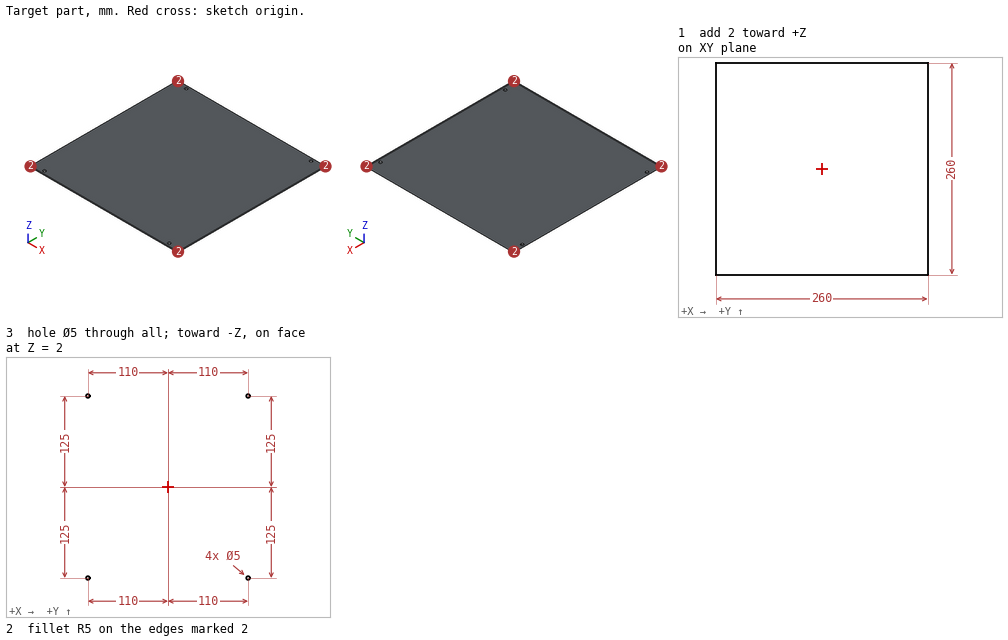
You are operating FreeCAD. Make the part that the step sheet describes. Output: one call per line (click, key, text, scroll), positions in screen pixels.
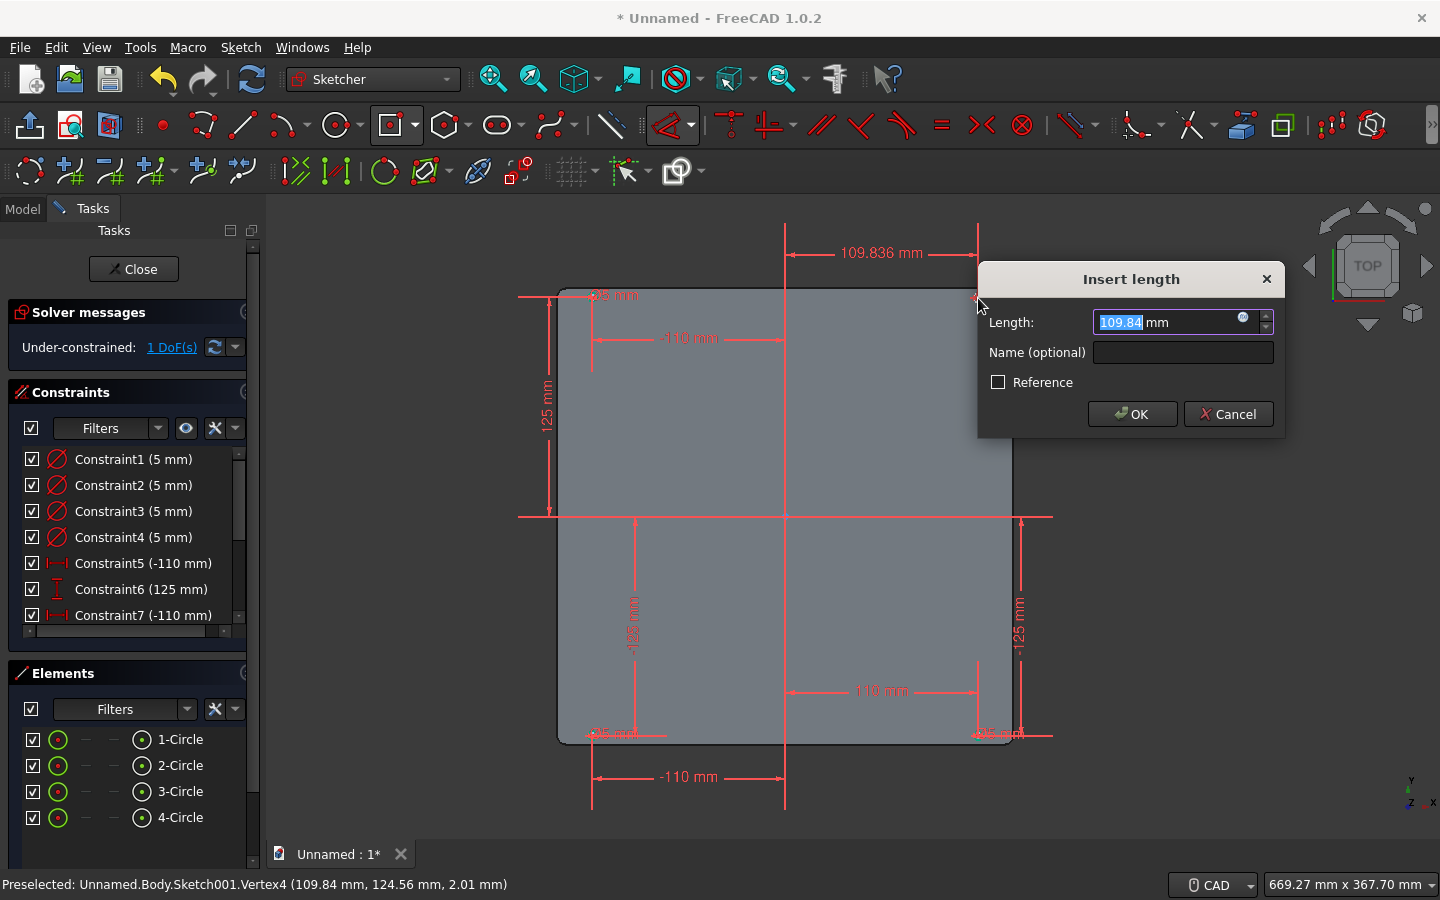
text(110)
key(Return)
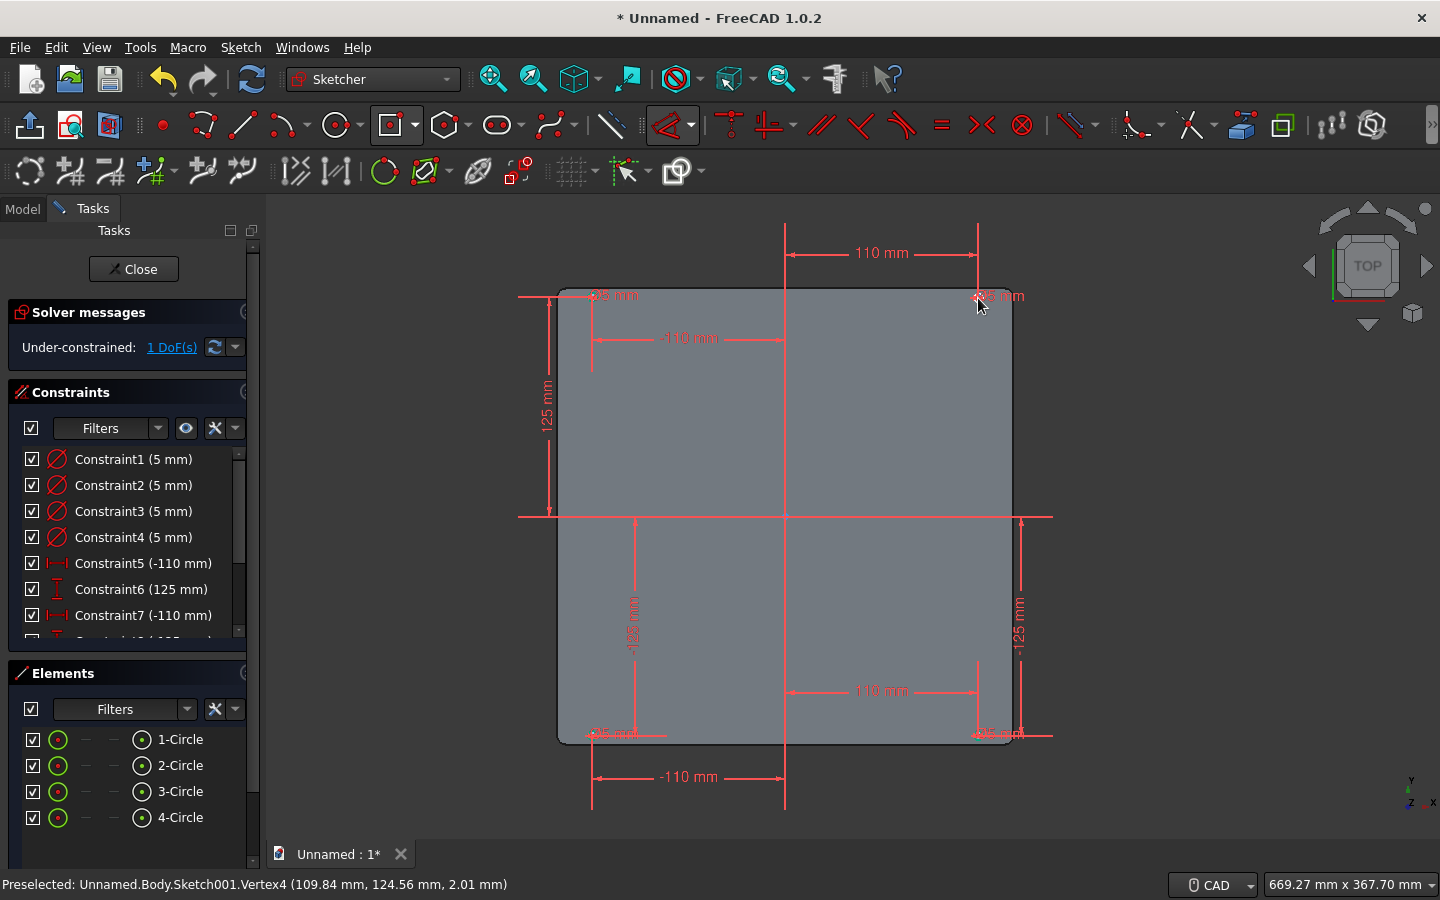
click(978, 298)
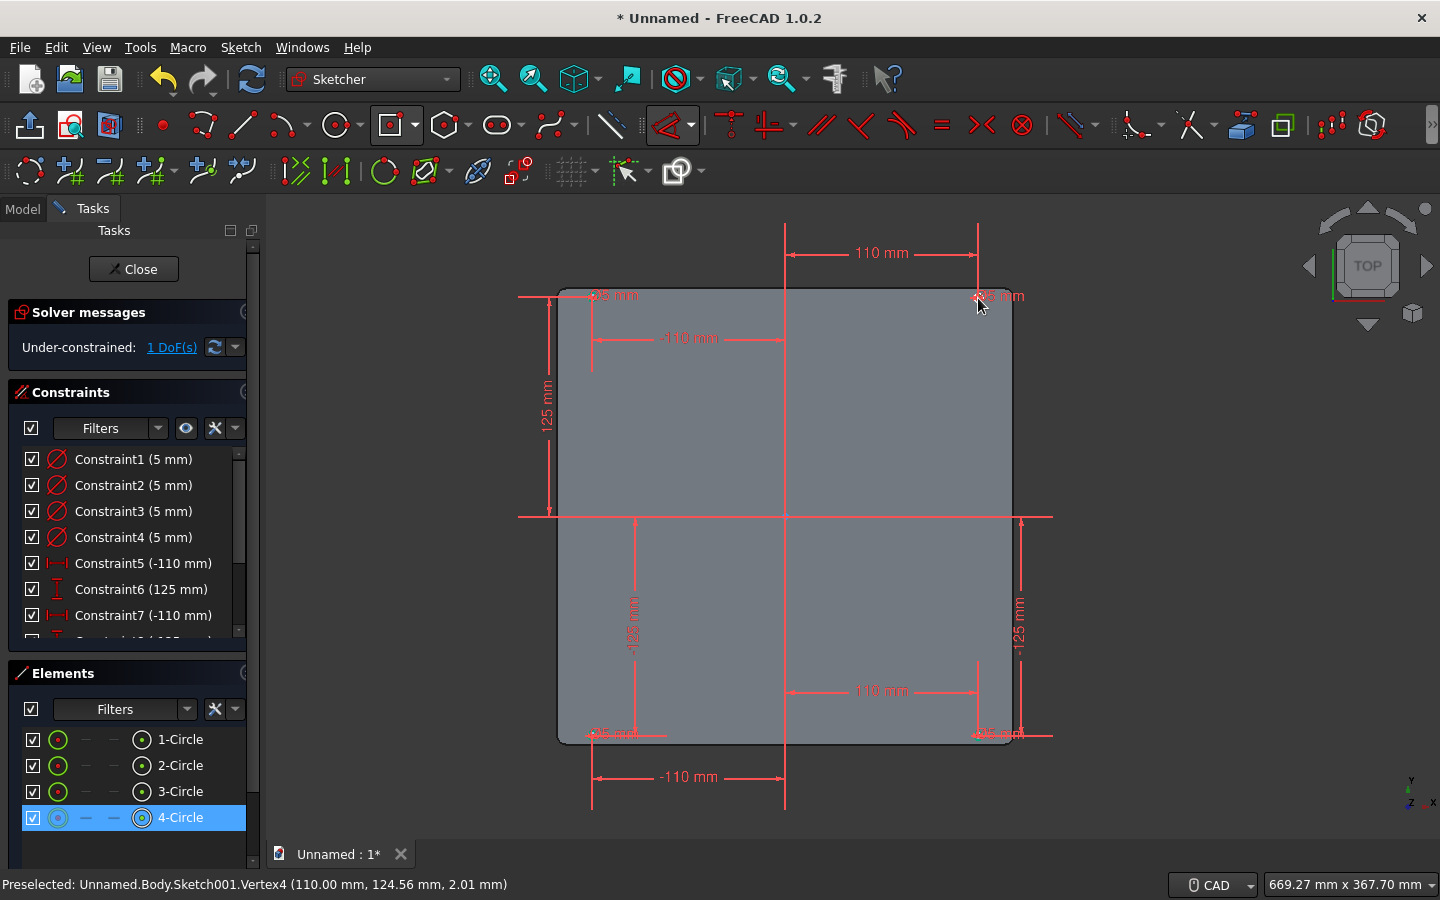
click(694, 126)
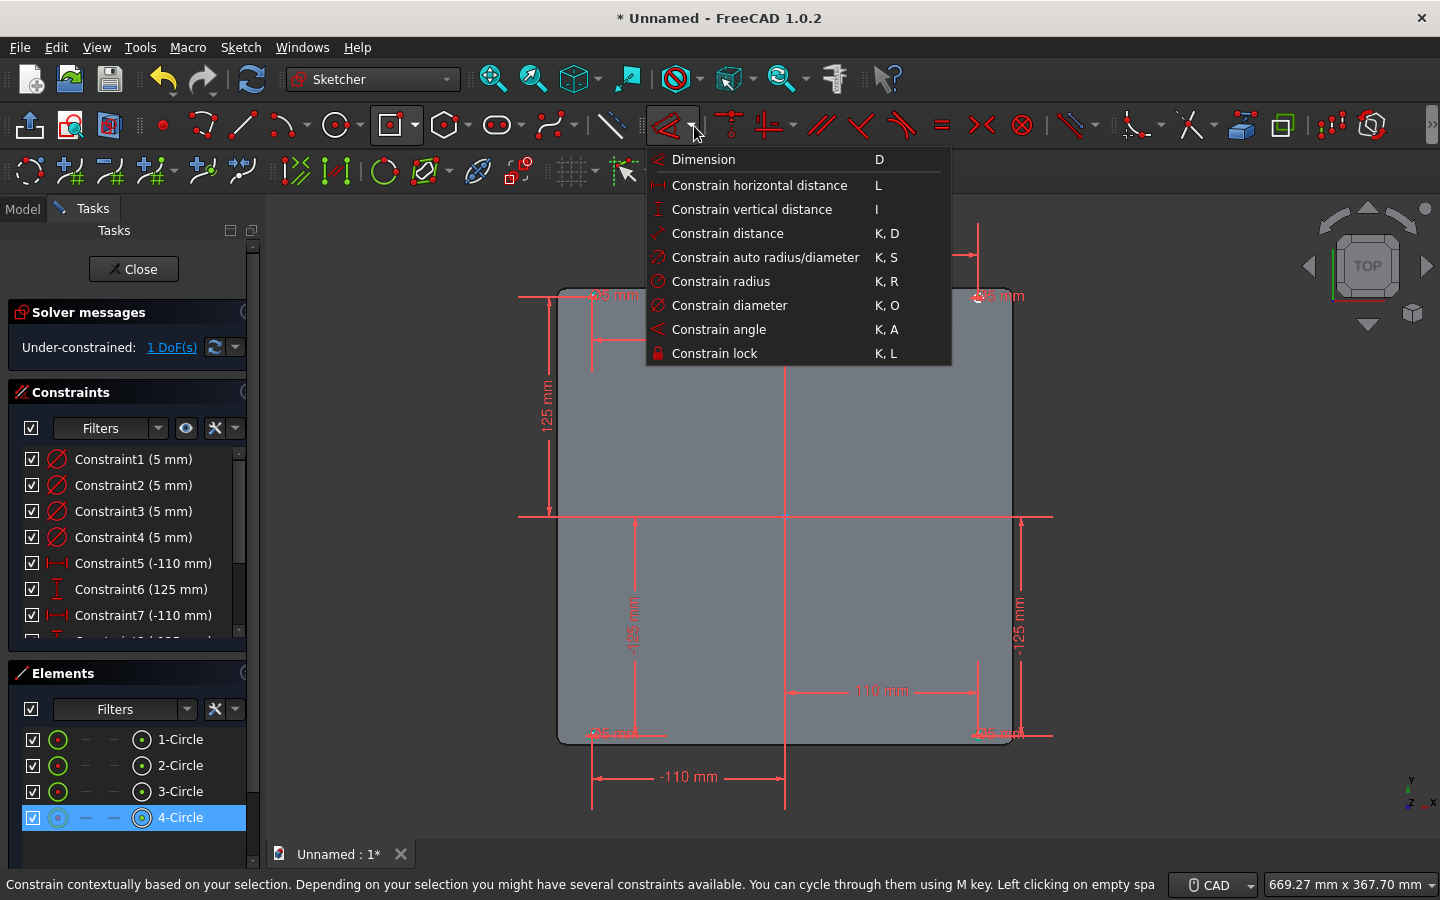
click(799, 209)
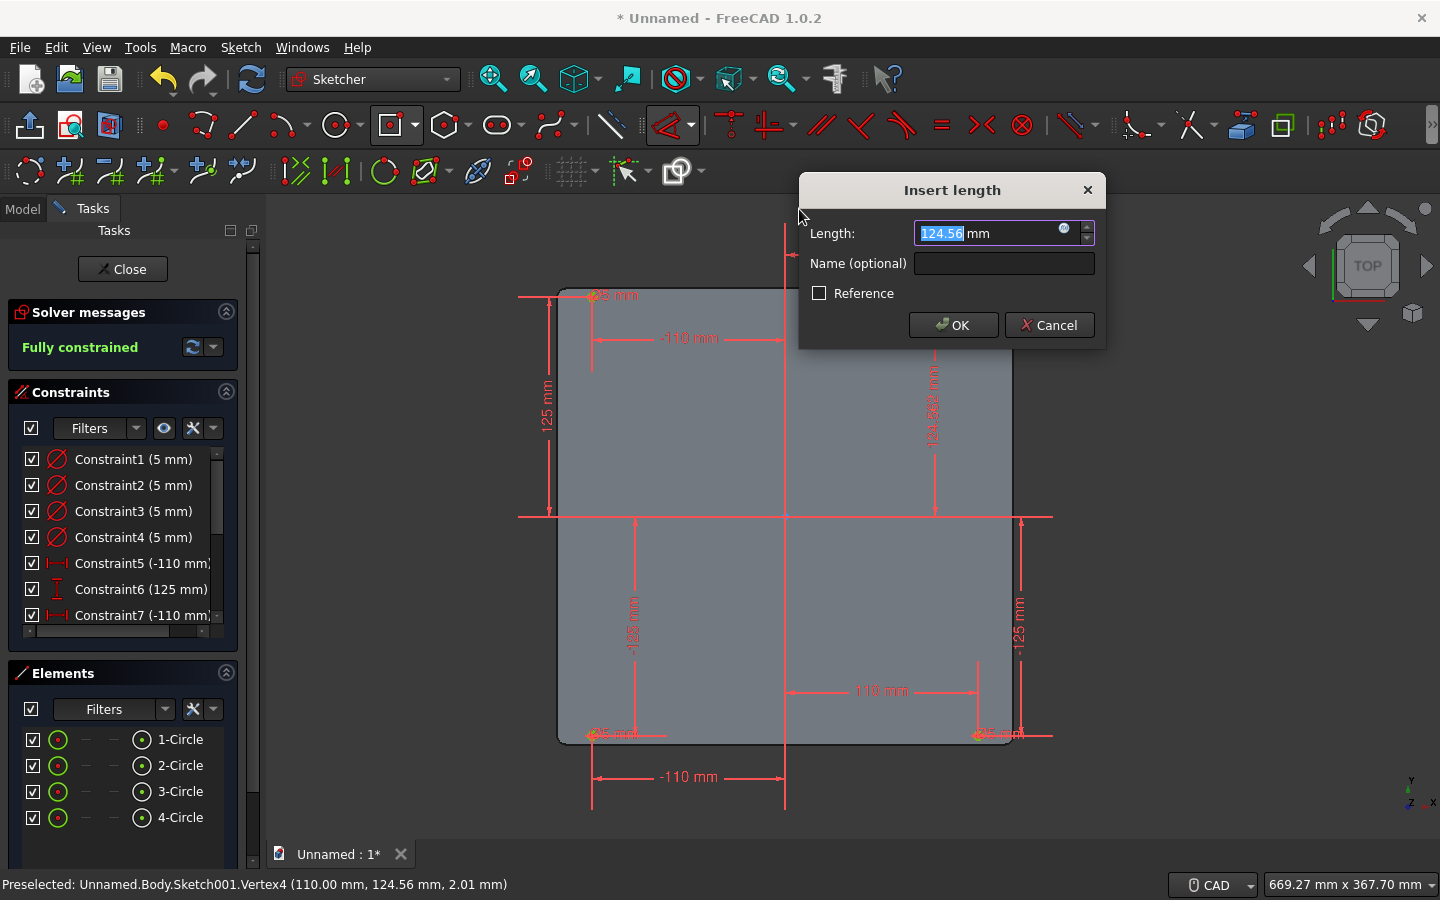
text(125)
key(Return)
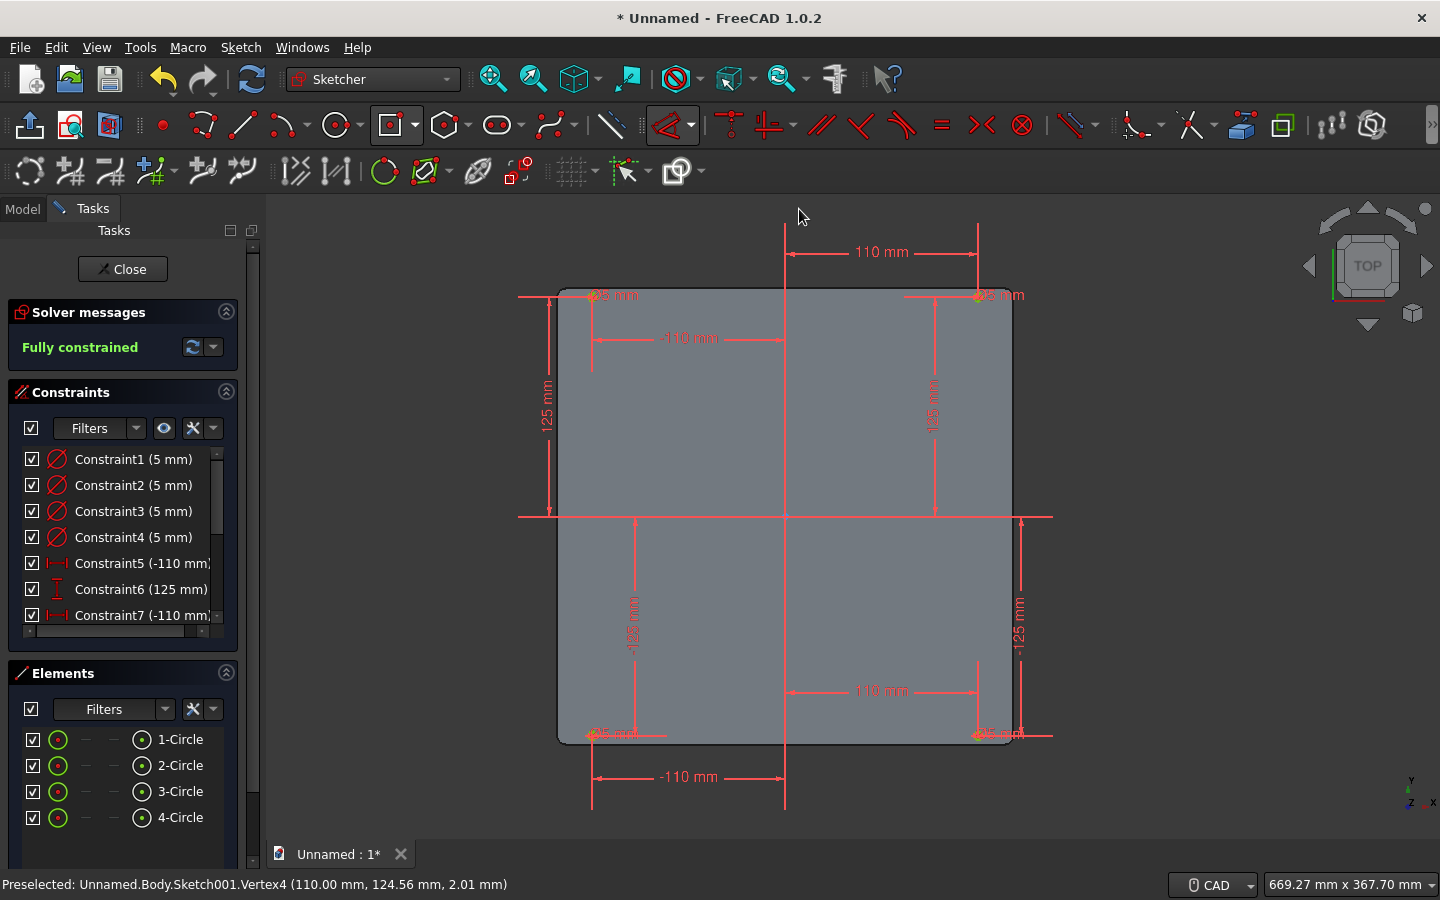
click(123, 269)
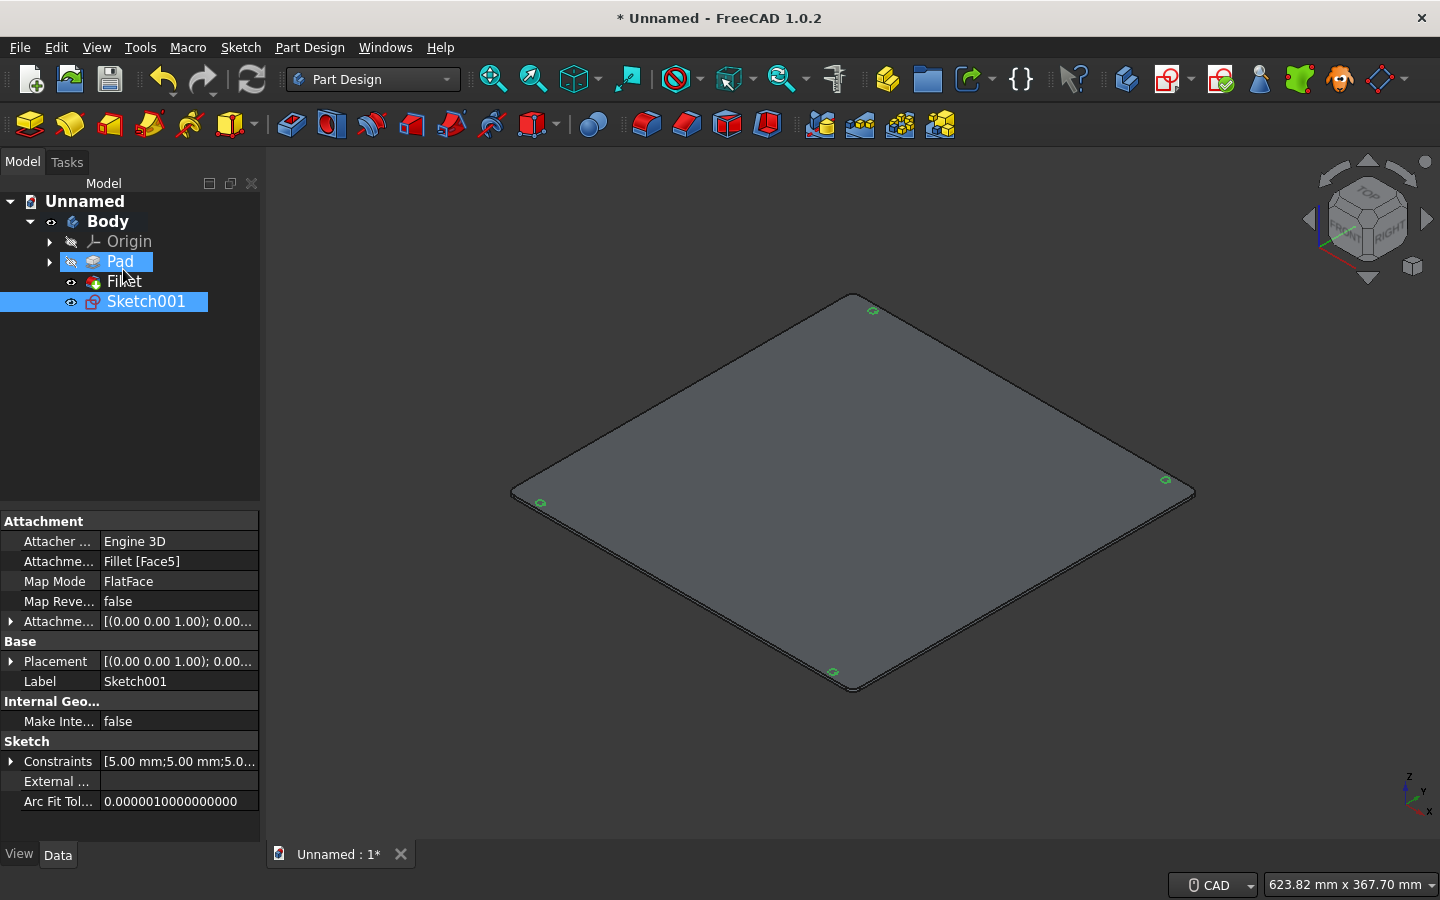
click(332, 124)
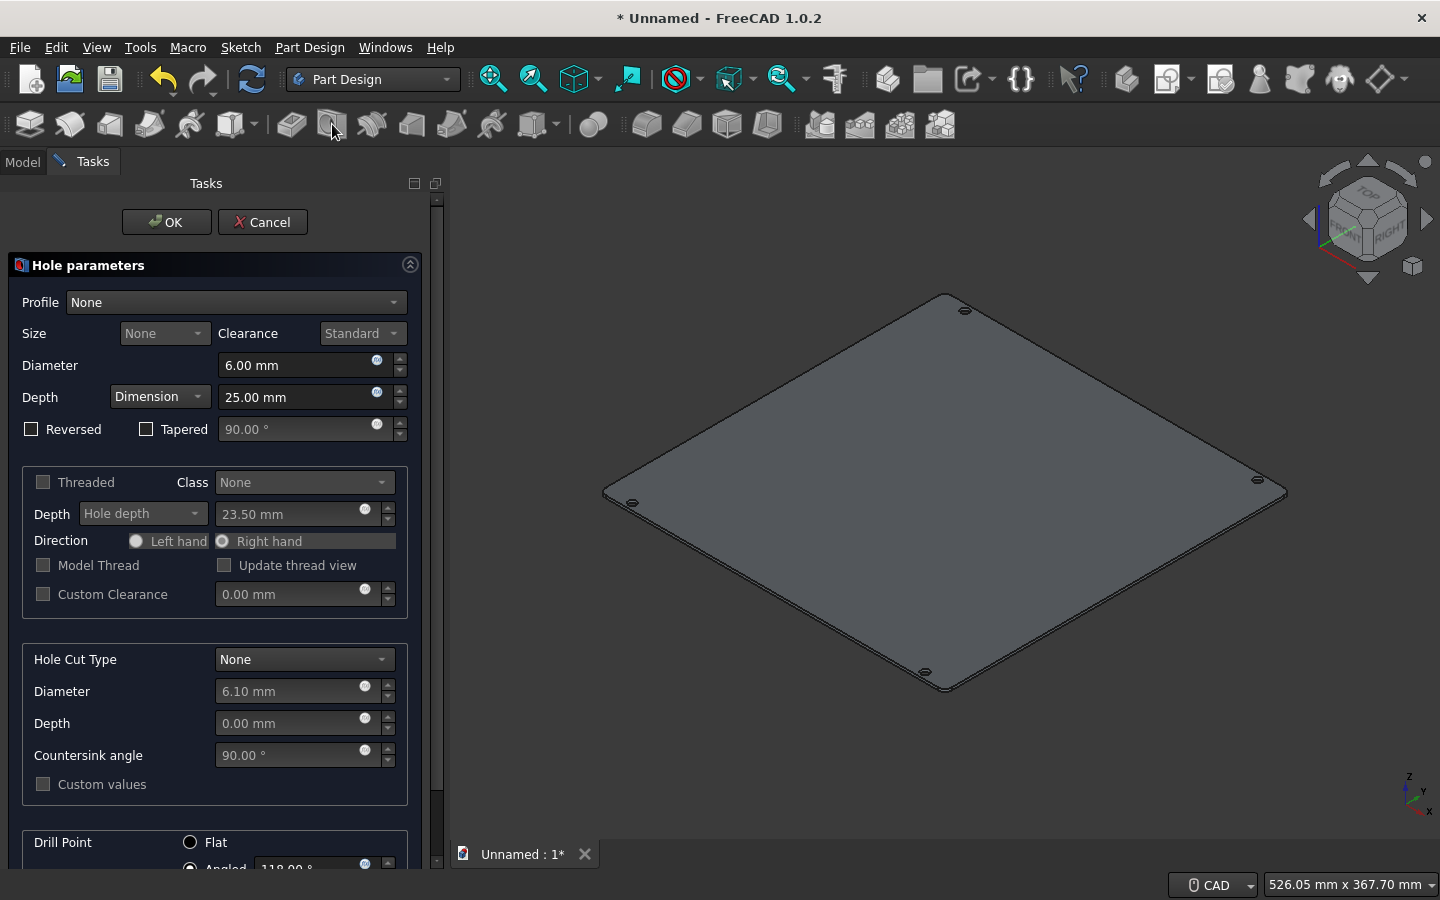
triple_click(305, 365)